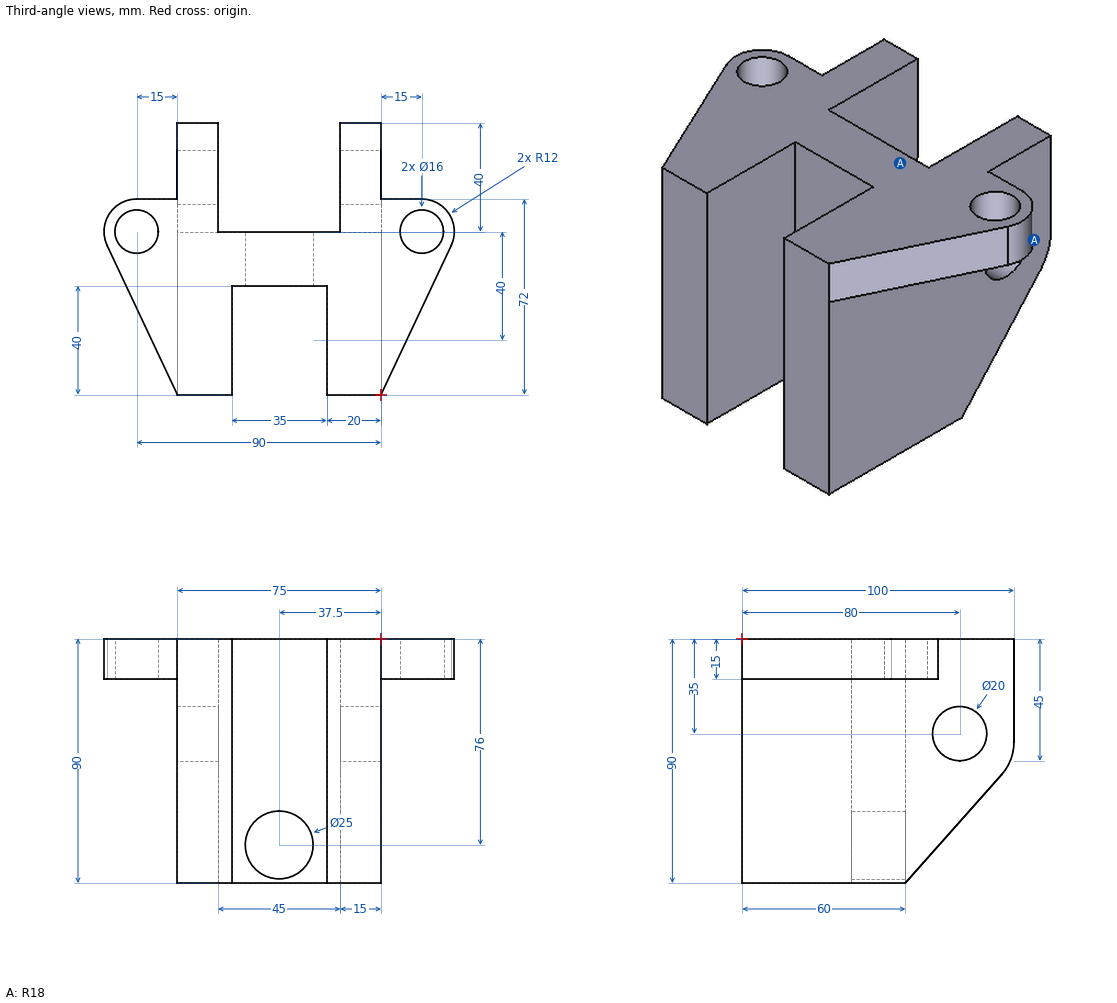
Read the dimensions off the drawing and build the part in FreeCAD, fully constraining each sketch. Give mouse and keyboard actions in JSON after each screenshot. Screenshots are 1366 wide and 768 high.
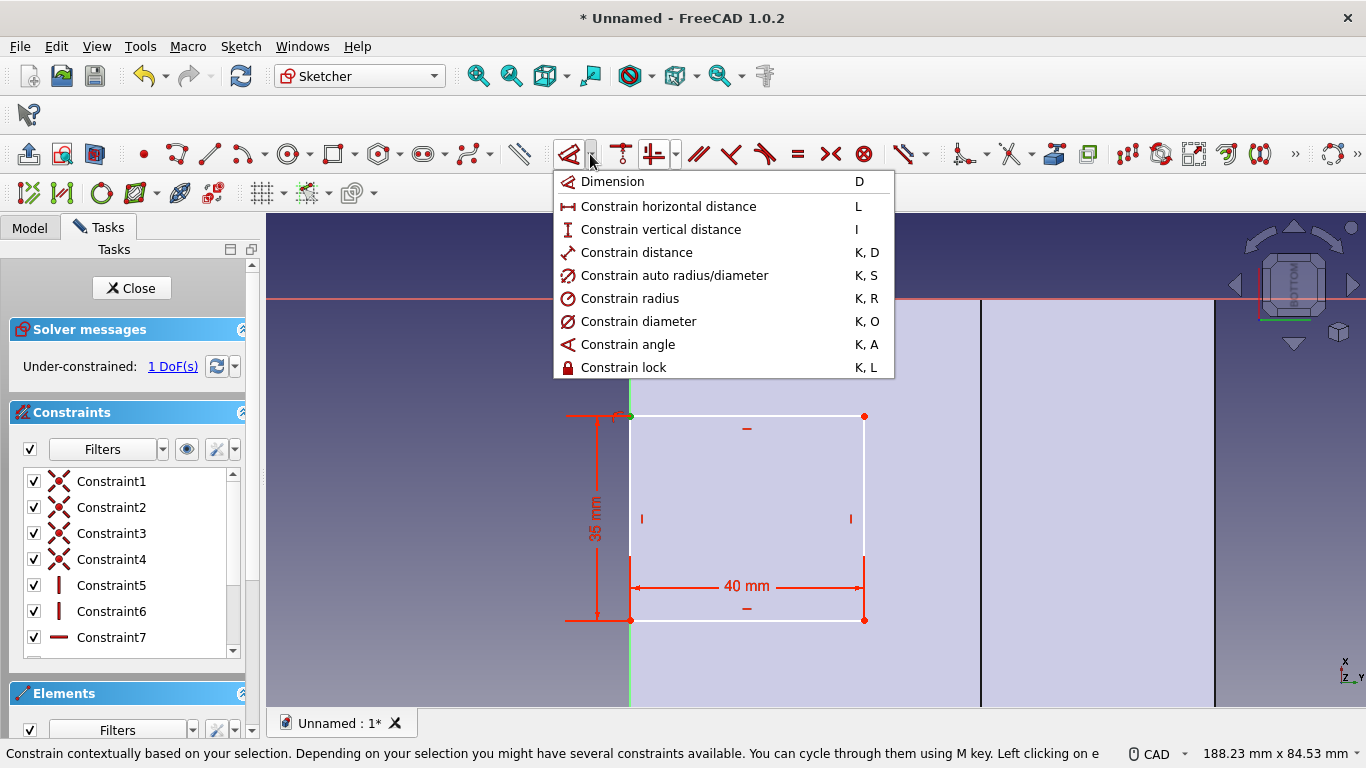
{"action": "left_click", "coordinate": [724, 230]}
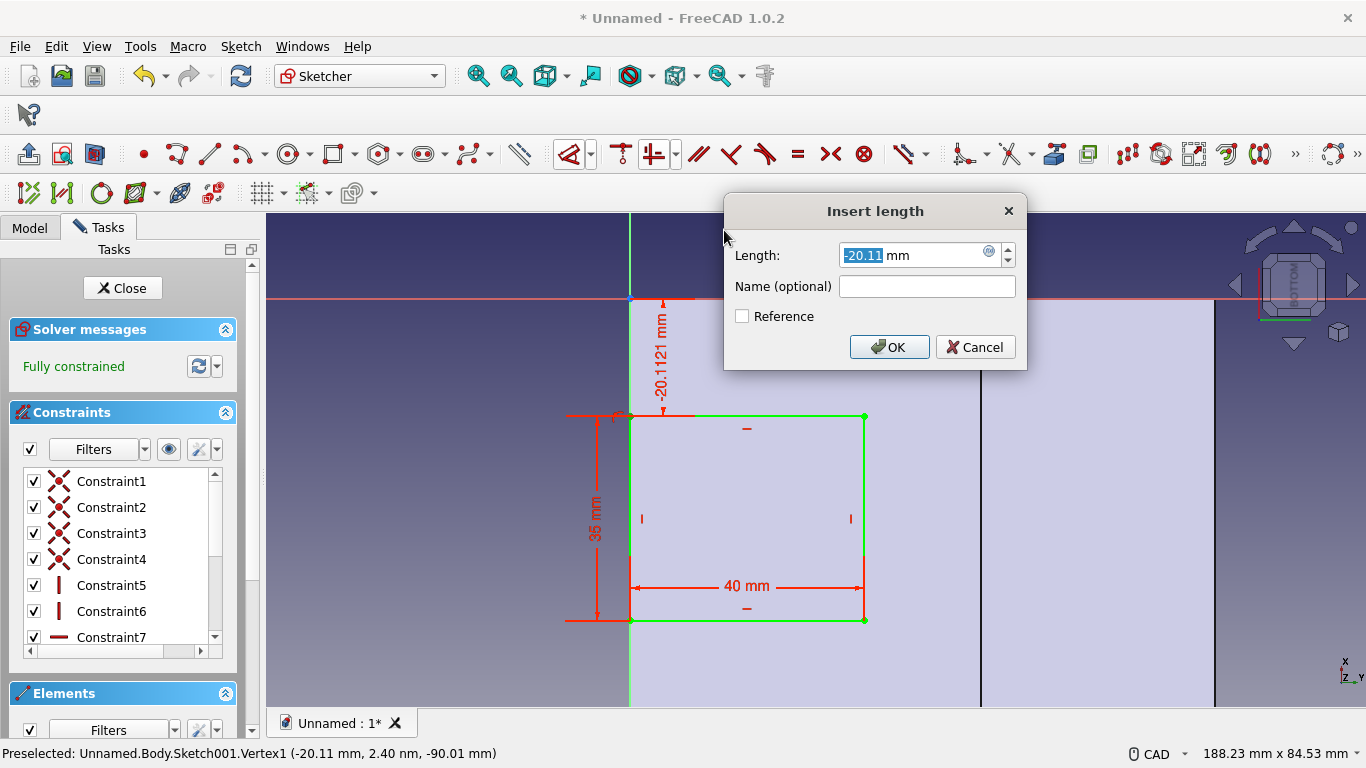
{"action": "type", "text": "-20"}
{"action": "key", "text": "Return"}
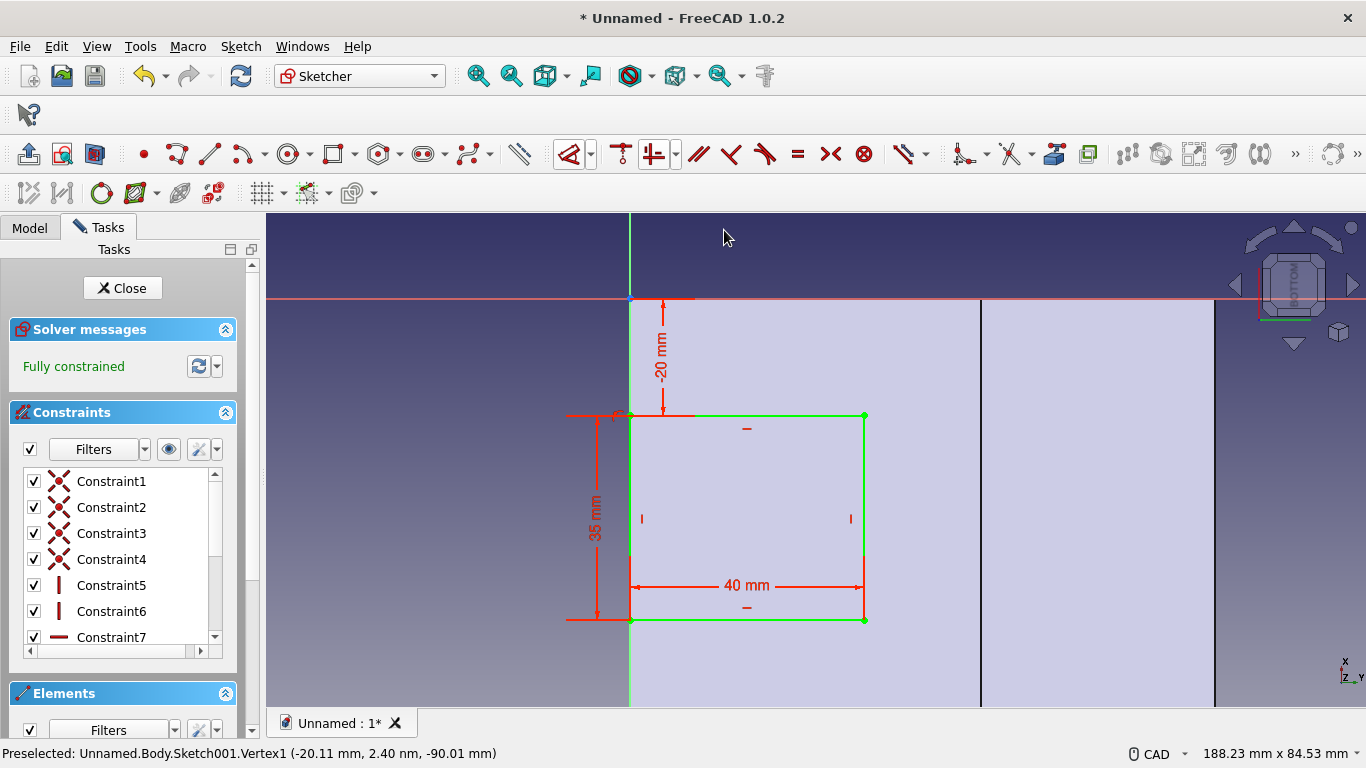
{"action": "left_click", "coordinate": [123, 288]}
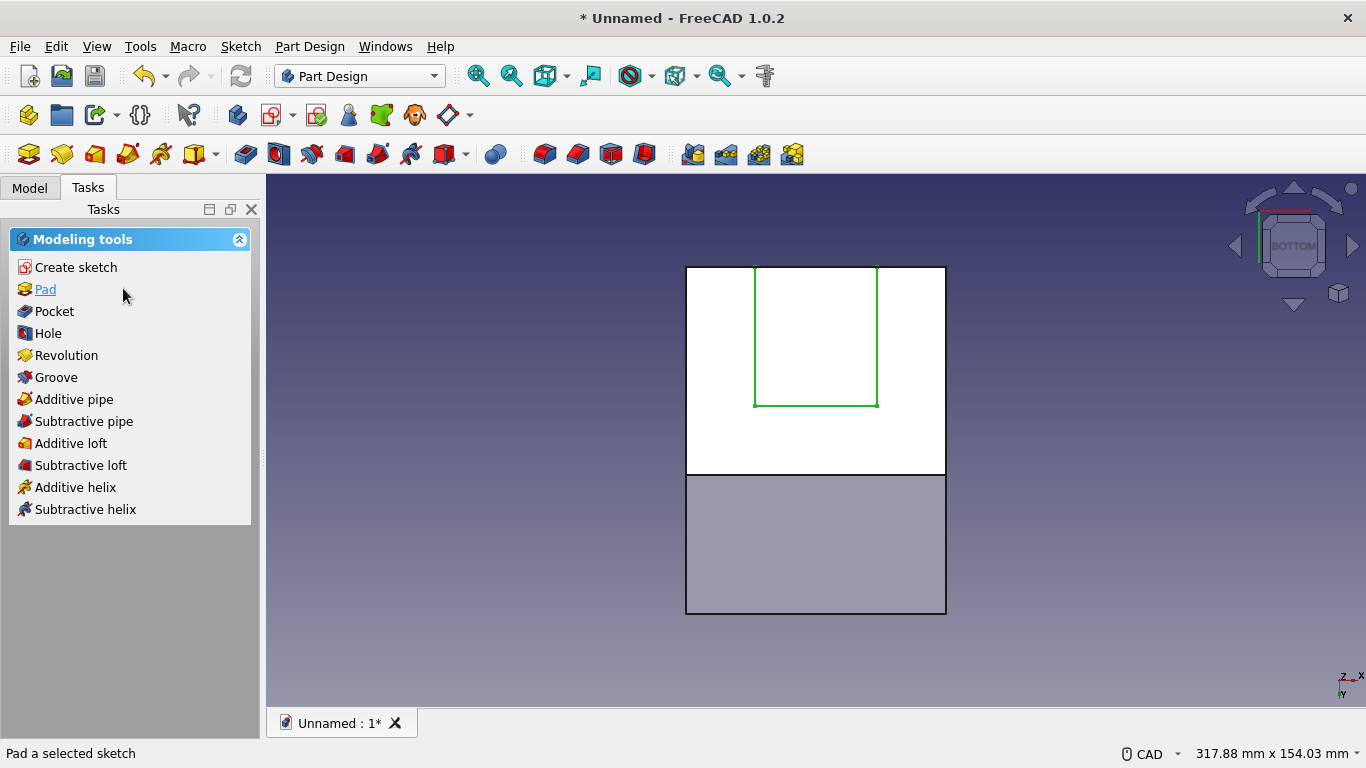
{"action": "left_click", "coordinate": [246, 154]}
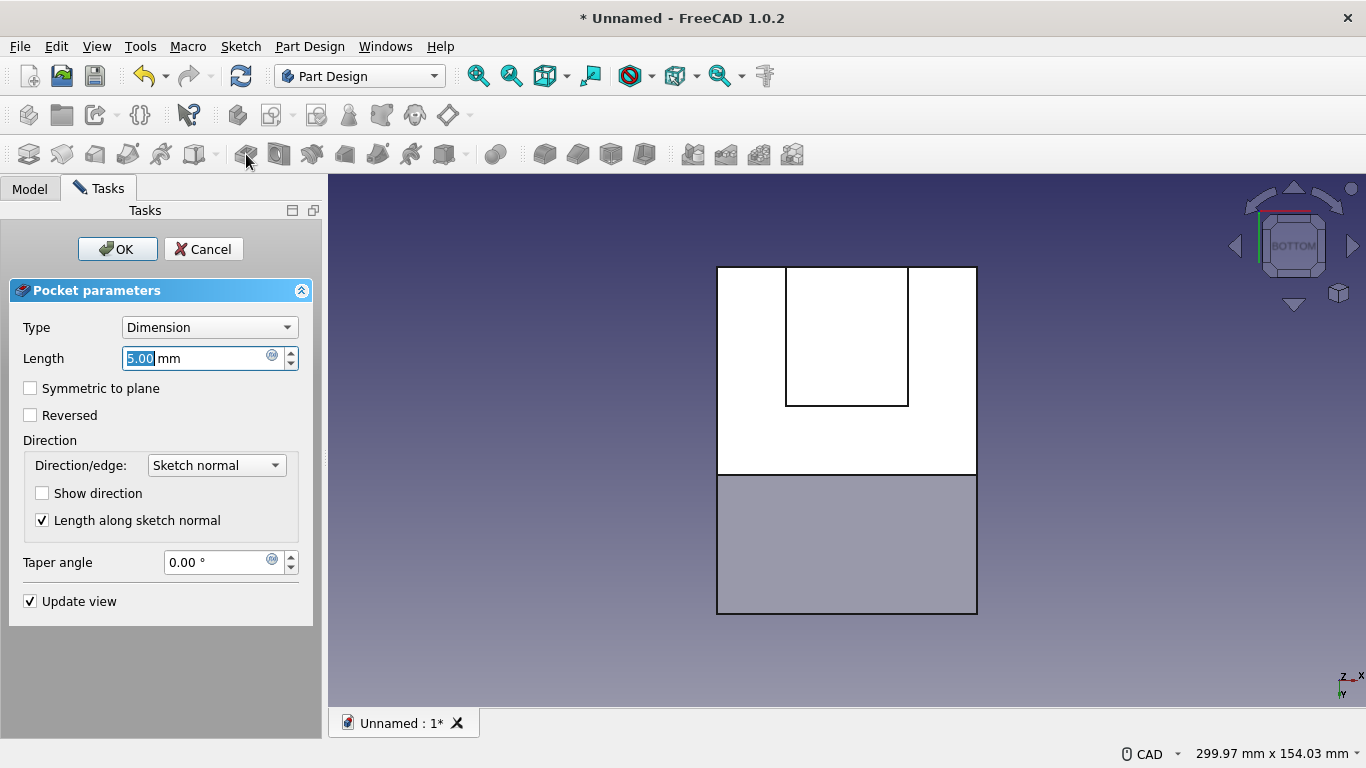
{"action": "left_click", "coordinate": [210, 328]}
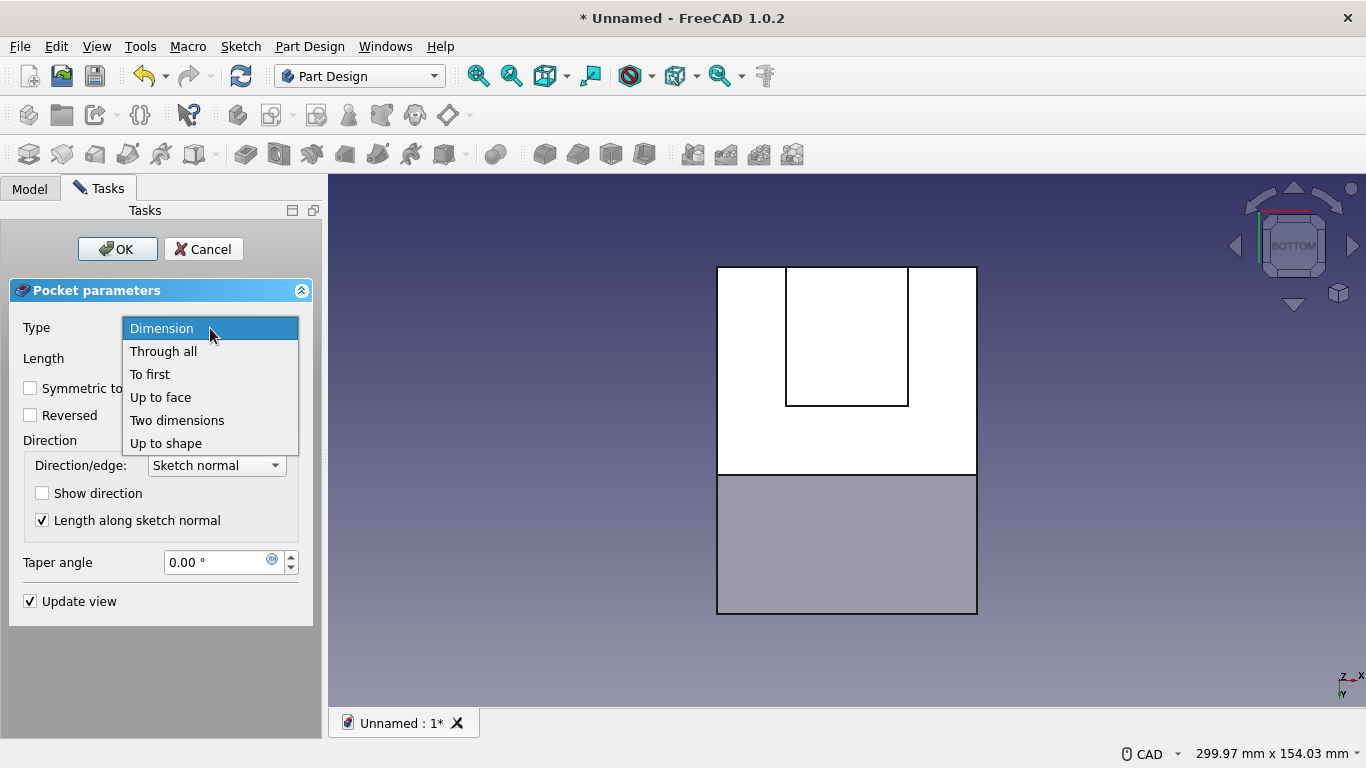
{"action": "left_click", "coordinate": [208, 352]}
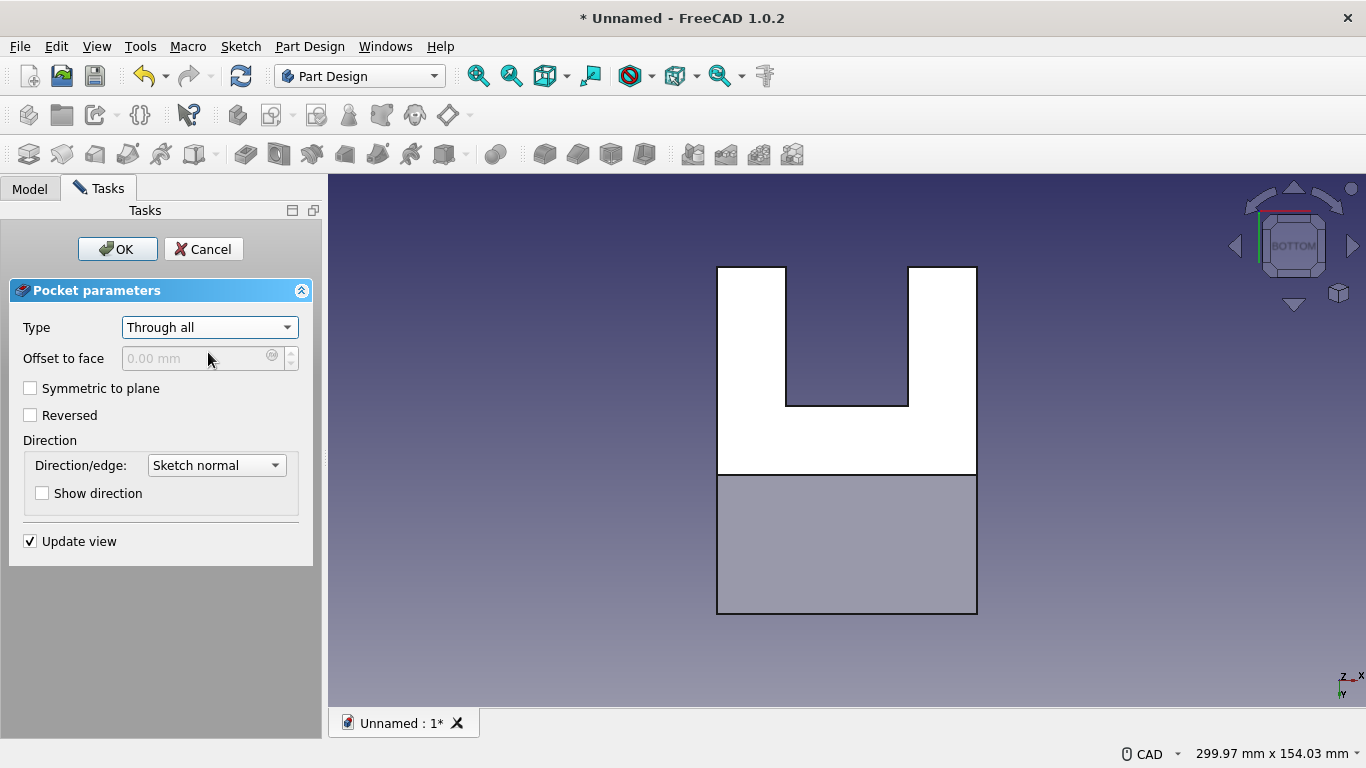
{"action": "left_click", "coordinate": [118, 249]}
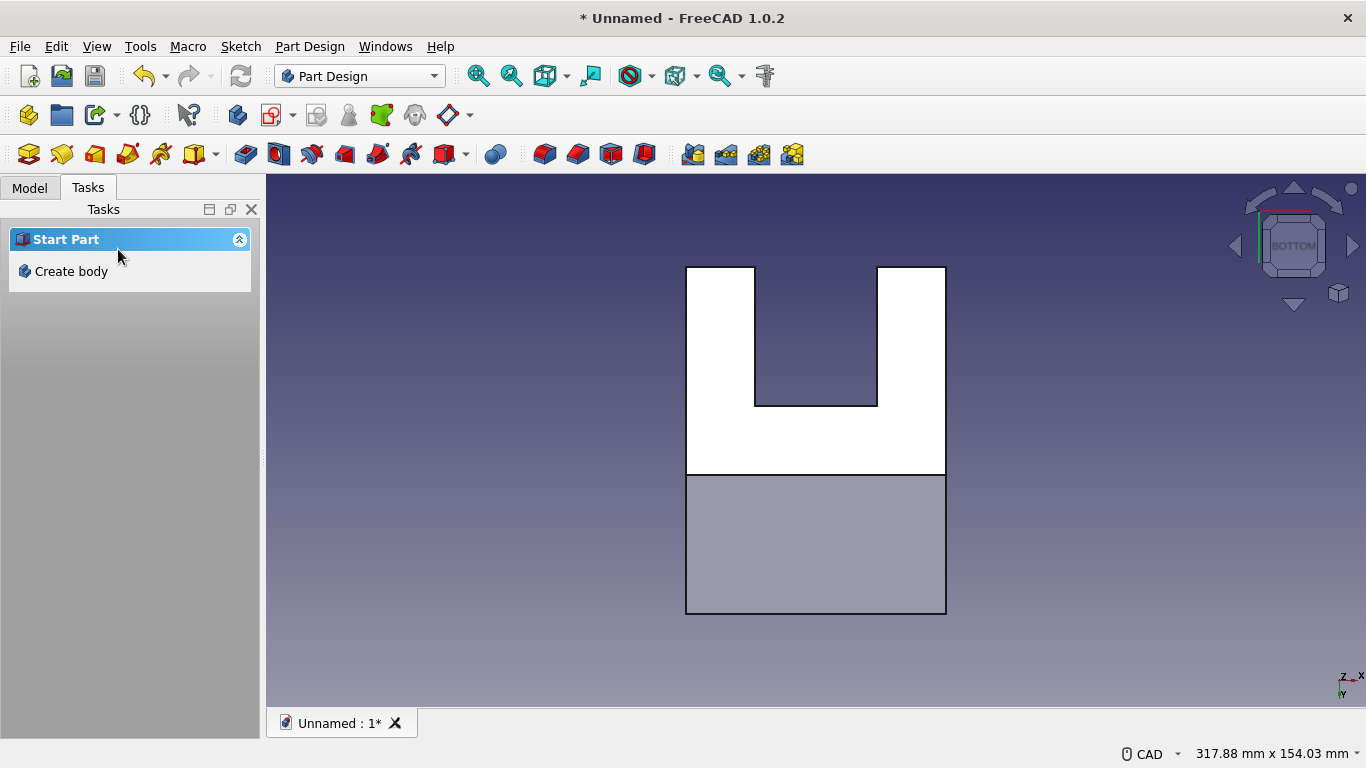
{"action": "key", "text": "4"}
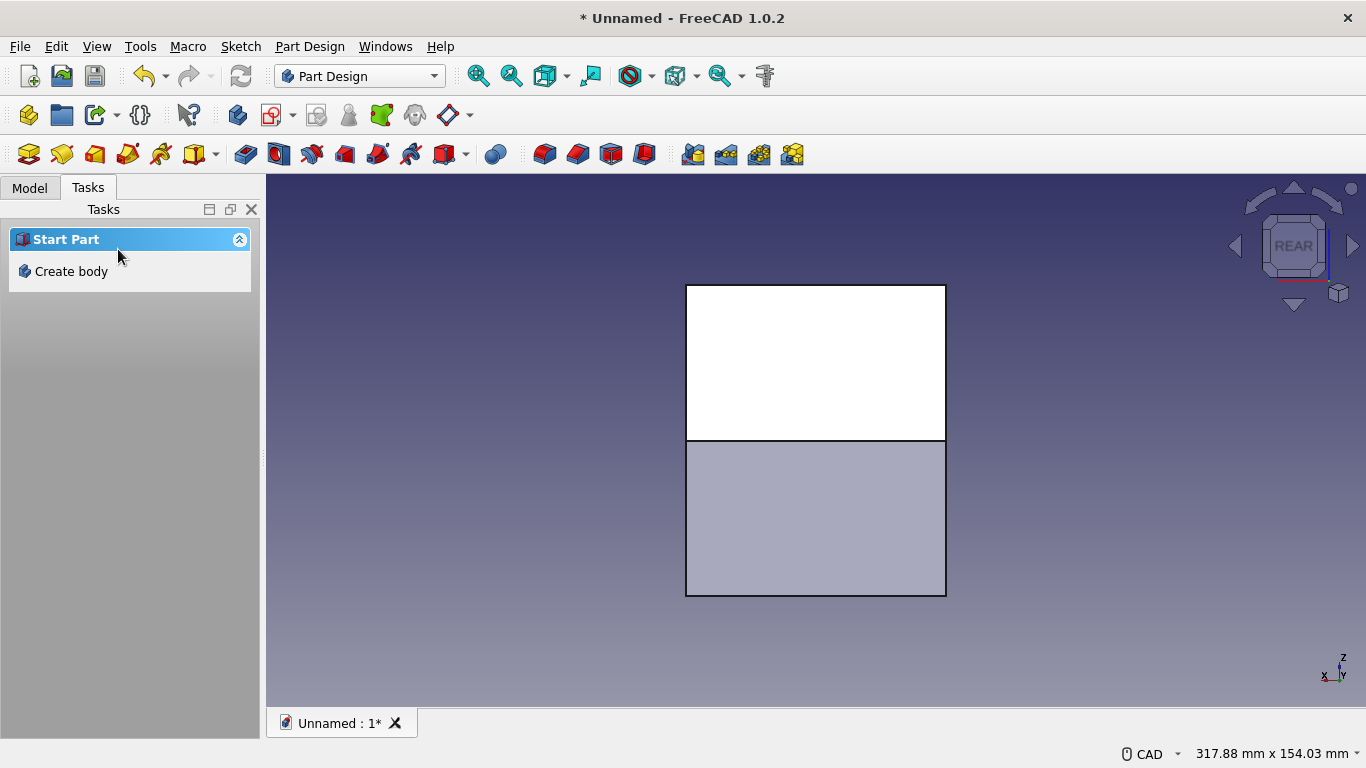
{"action": "left_click", "coordinate": [779, 362]}